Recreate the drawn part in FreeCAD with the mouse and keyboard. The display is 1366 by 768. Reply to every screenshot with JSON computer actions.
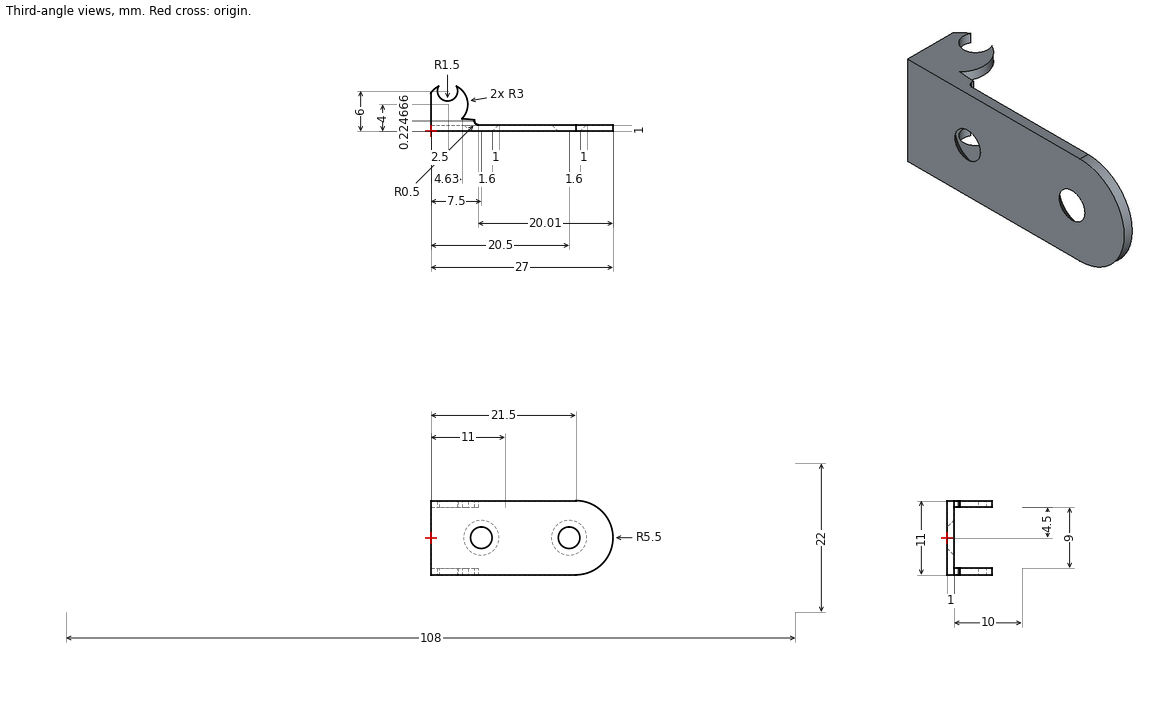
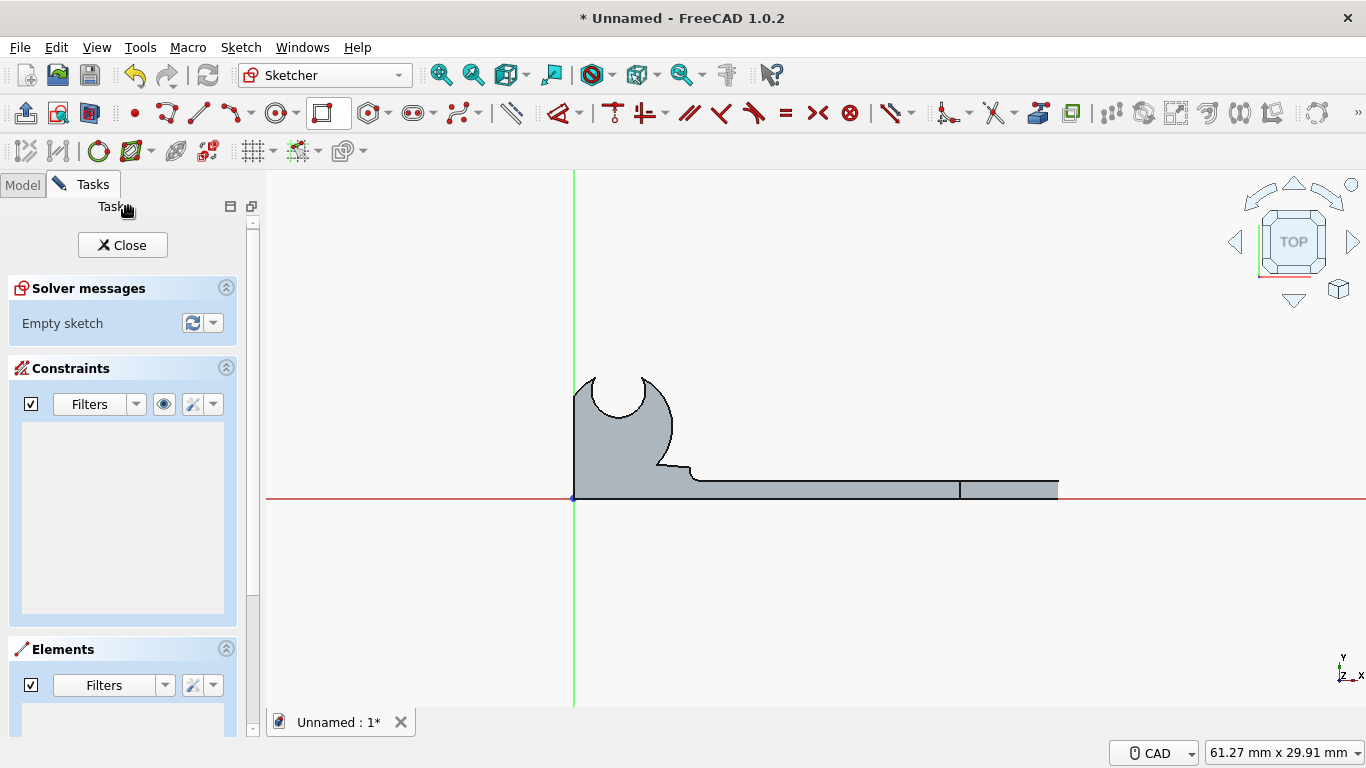
{"action": "key", "text": "q s"}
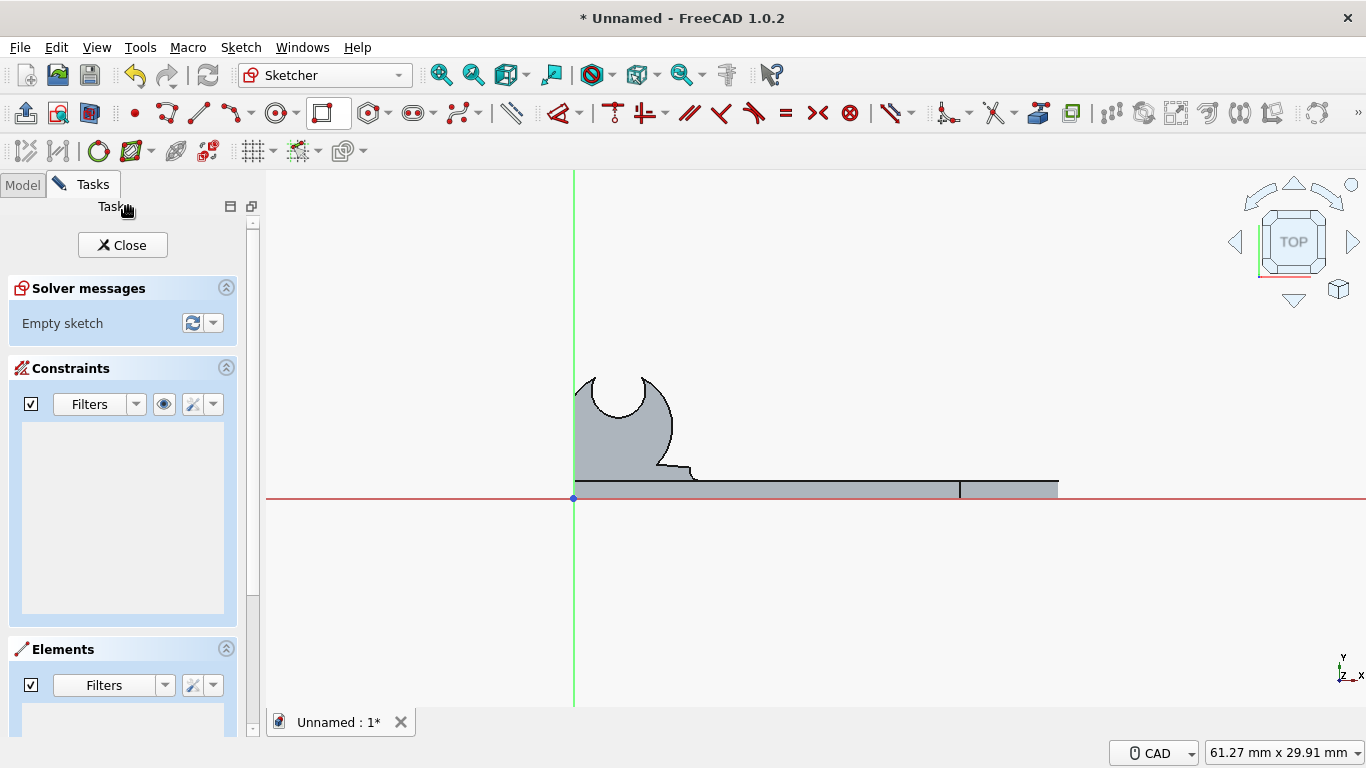
{"action": "scroll", "coordinate": [730, 490], "scroll_direction": "up", "scroll_amount": 13}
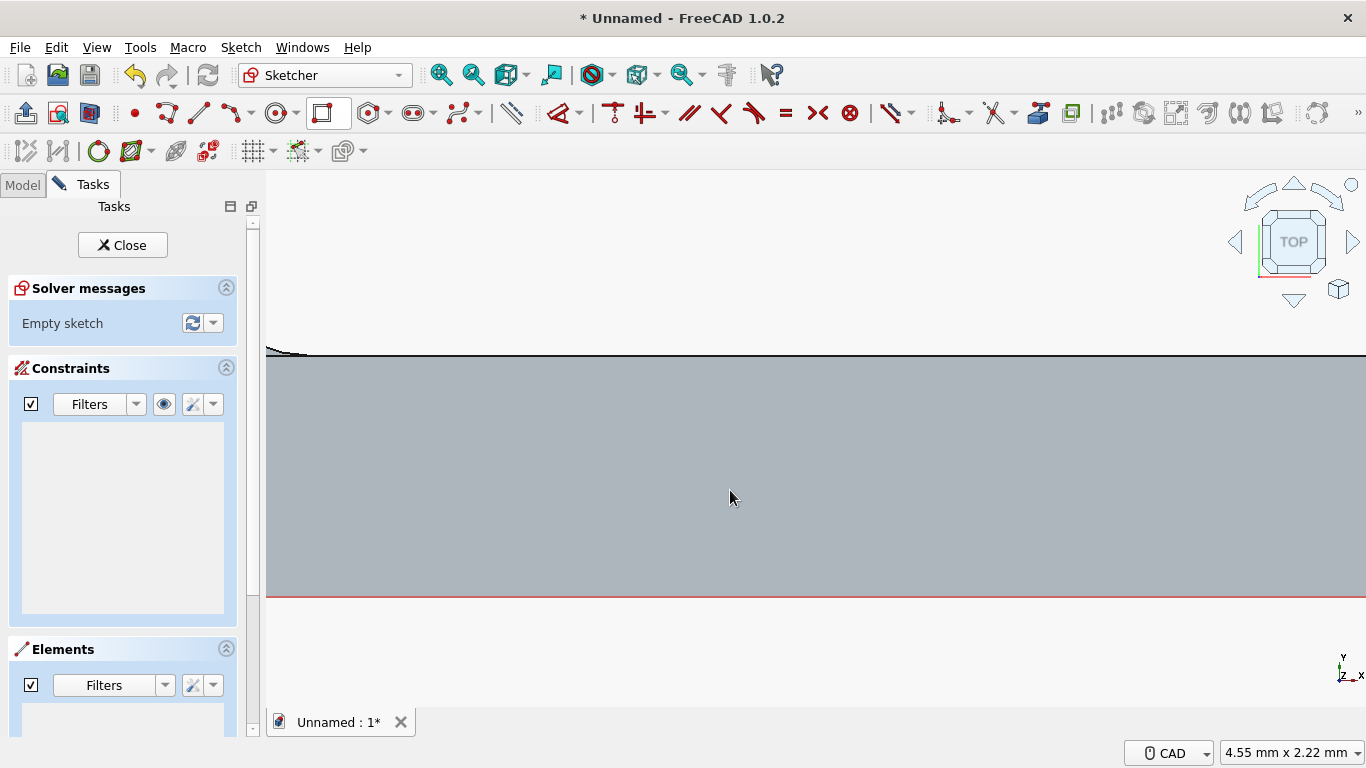
{"action": "left_click", "coordinate": [168, 114]}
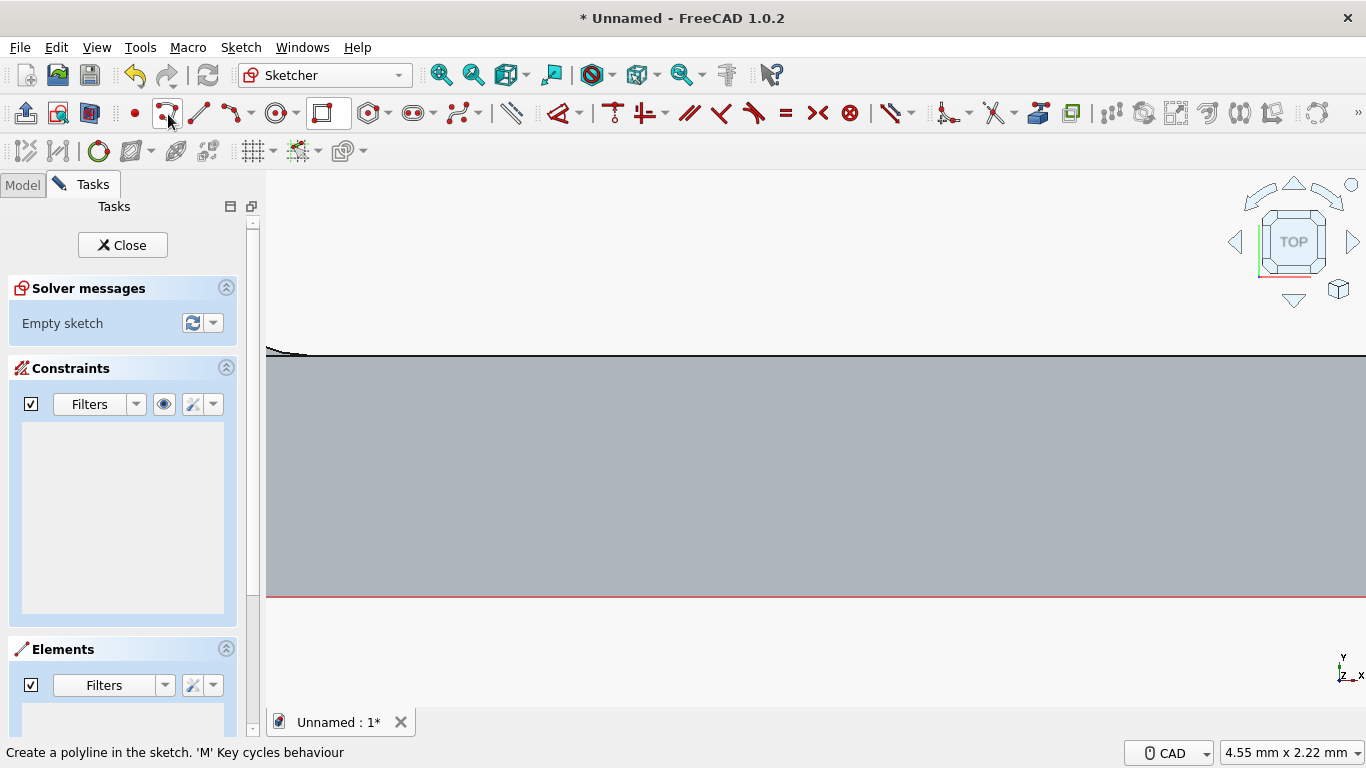
{"action": "left_click", "coordinate": [432, 597]}
{"action": "left_click", "coordinate": [819, 588]}
{"action": "left_click", "coordinate": [1061, 356]}
{"action": "left_click", "coordinate": [432, 356]}
{"action": "left_click", "coordinate": [432, 597]}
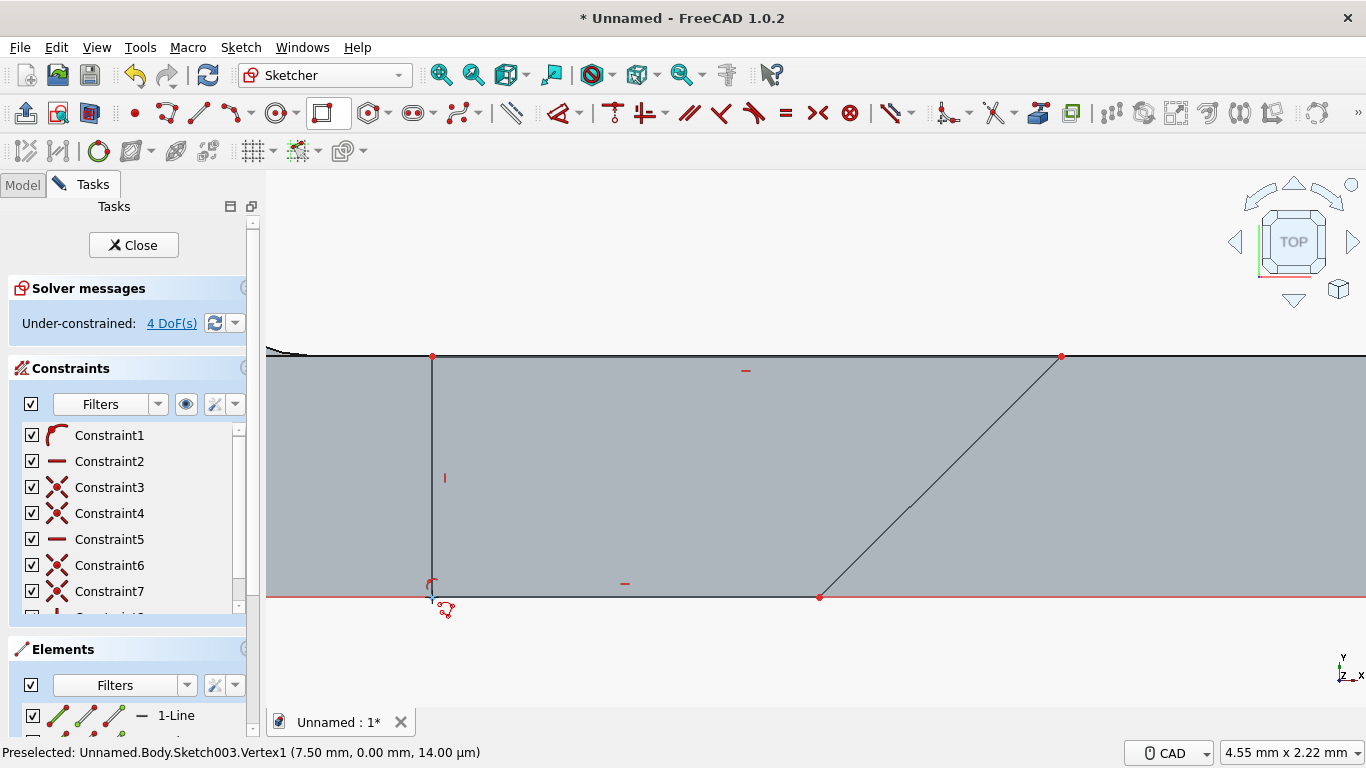
{"action": "key", "text": "g l"}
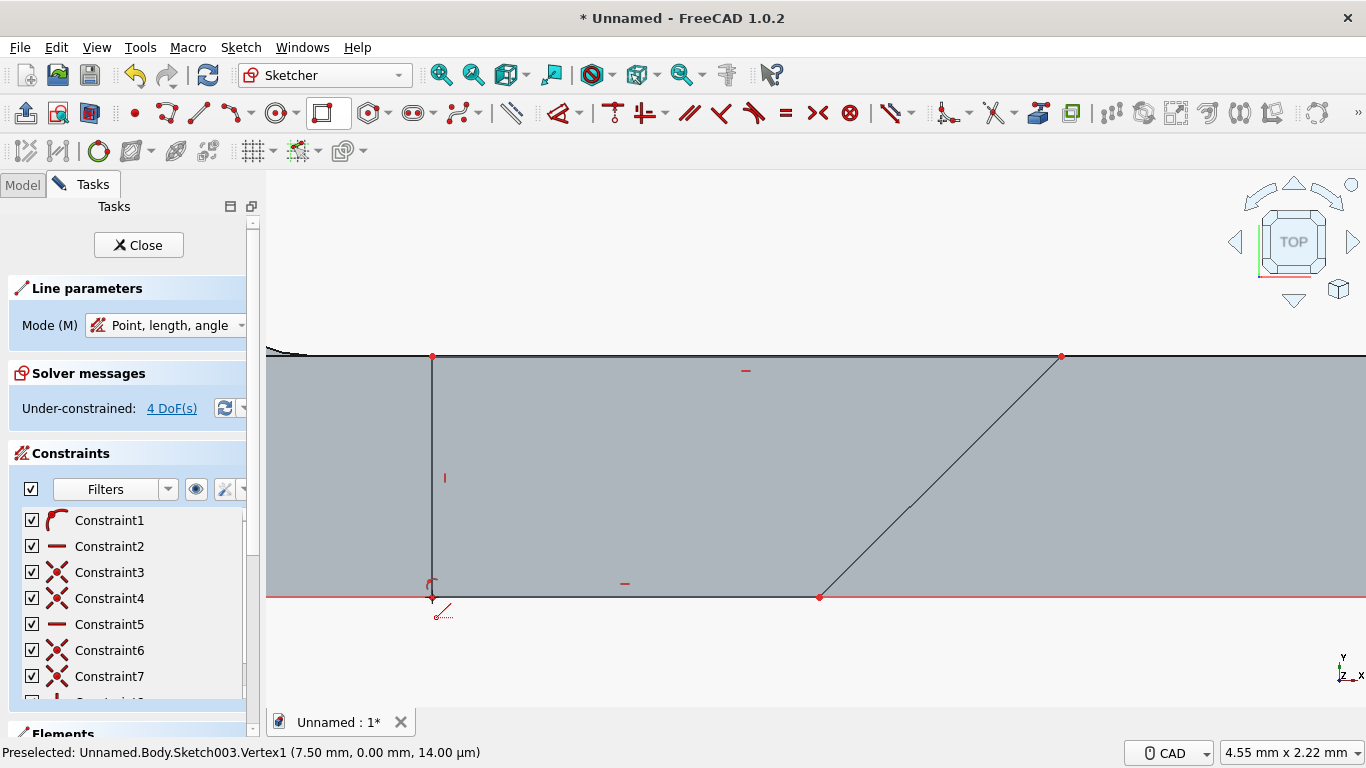
{"action": "left_click", "coordinate": [432, 331]}
{"action": "left_click", "coordinate": [432, 255]}
{"action": "key", "text": "Escape"}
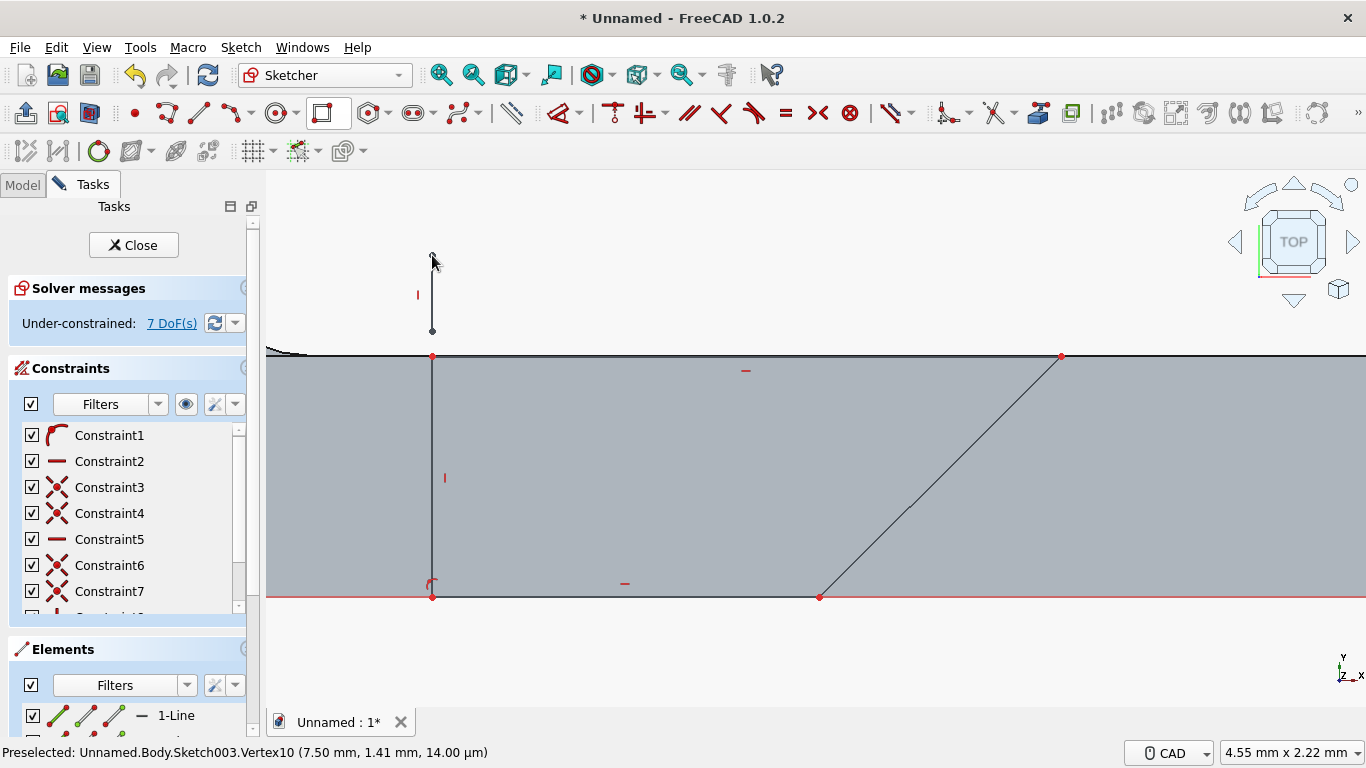
{"action": "left_click", "coordinate": [432, 309]}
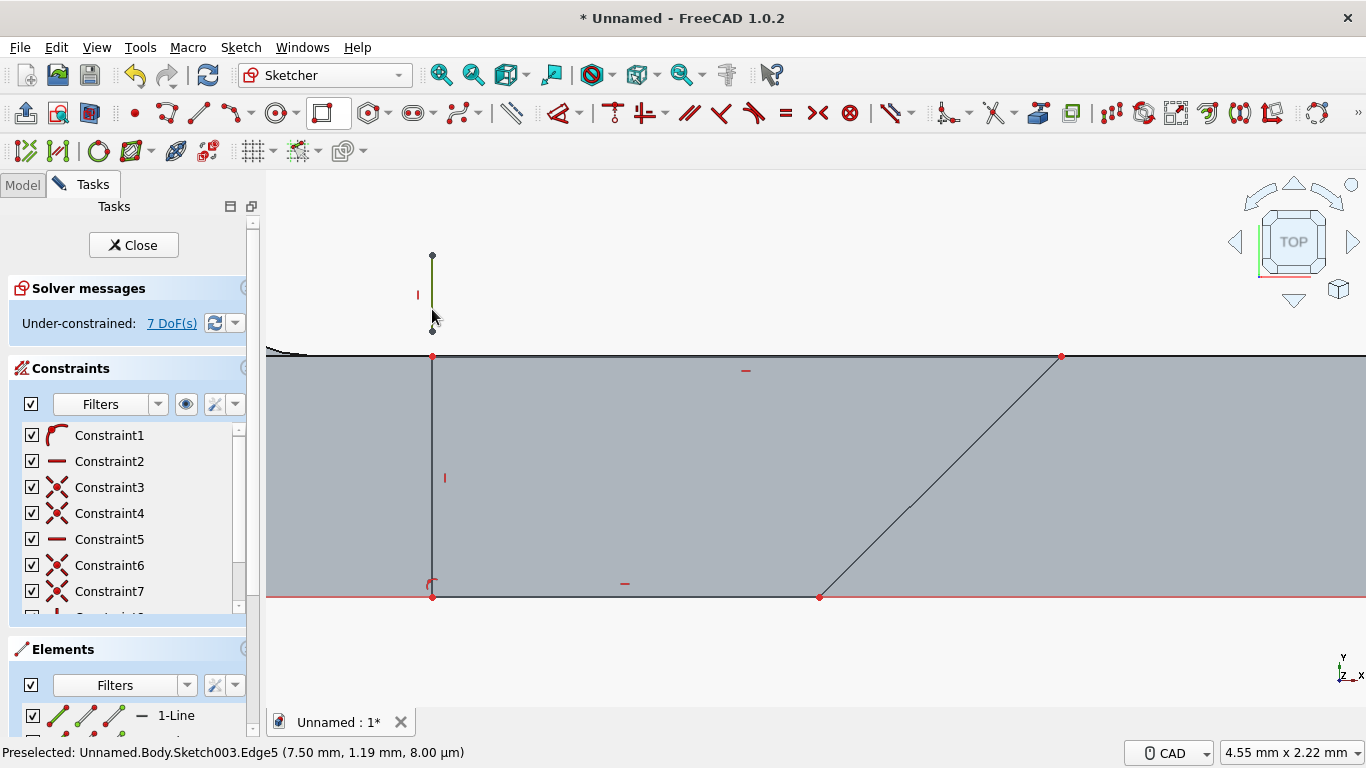
{"action": "left_click", "coordinate": [512, 114]}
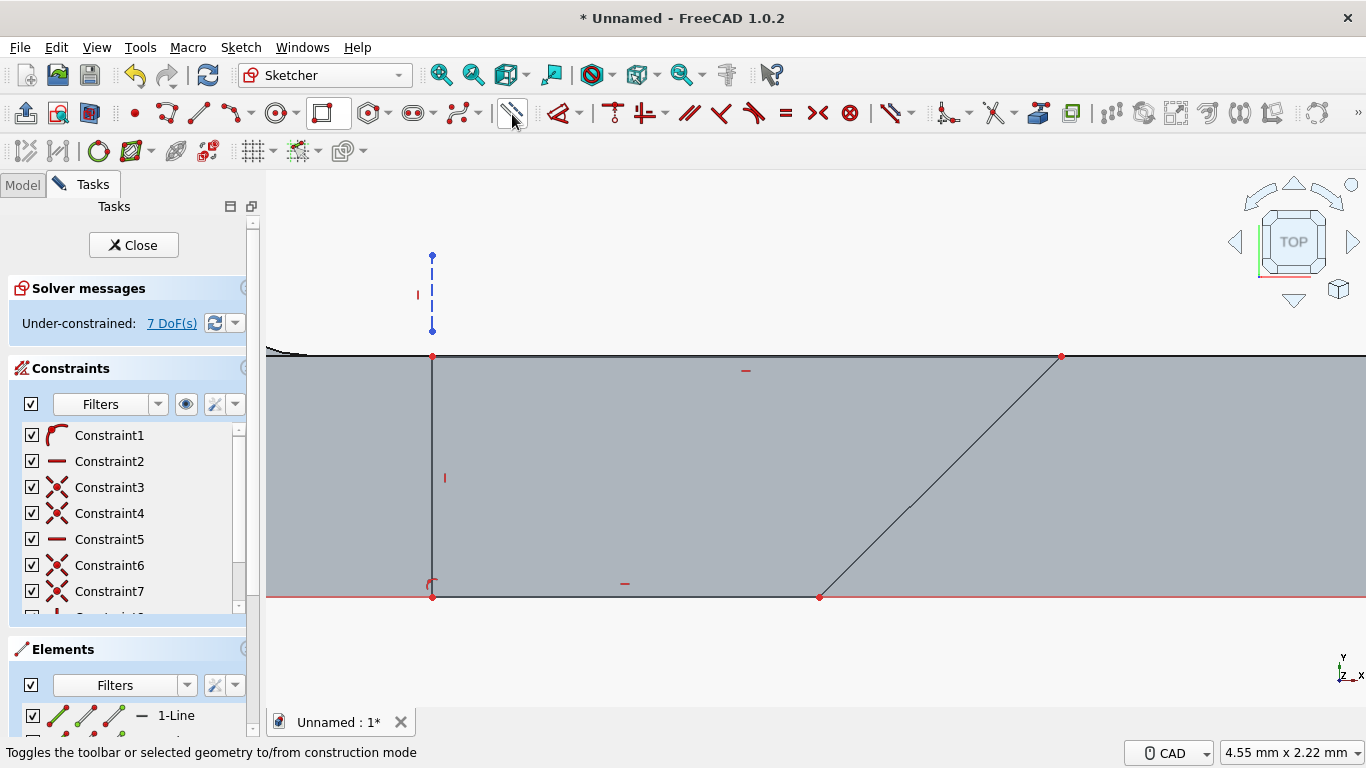
{"action": "left_click", "coordinate": [558, 114]}